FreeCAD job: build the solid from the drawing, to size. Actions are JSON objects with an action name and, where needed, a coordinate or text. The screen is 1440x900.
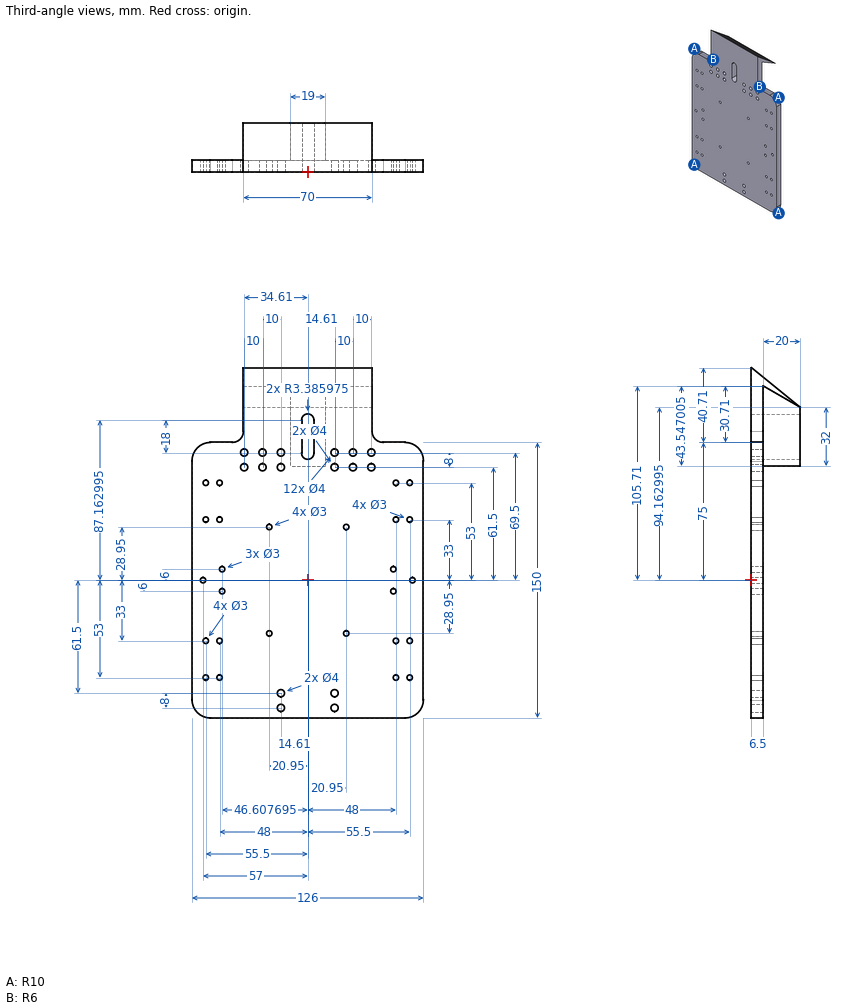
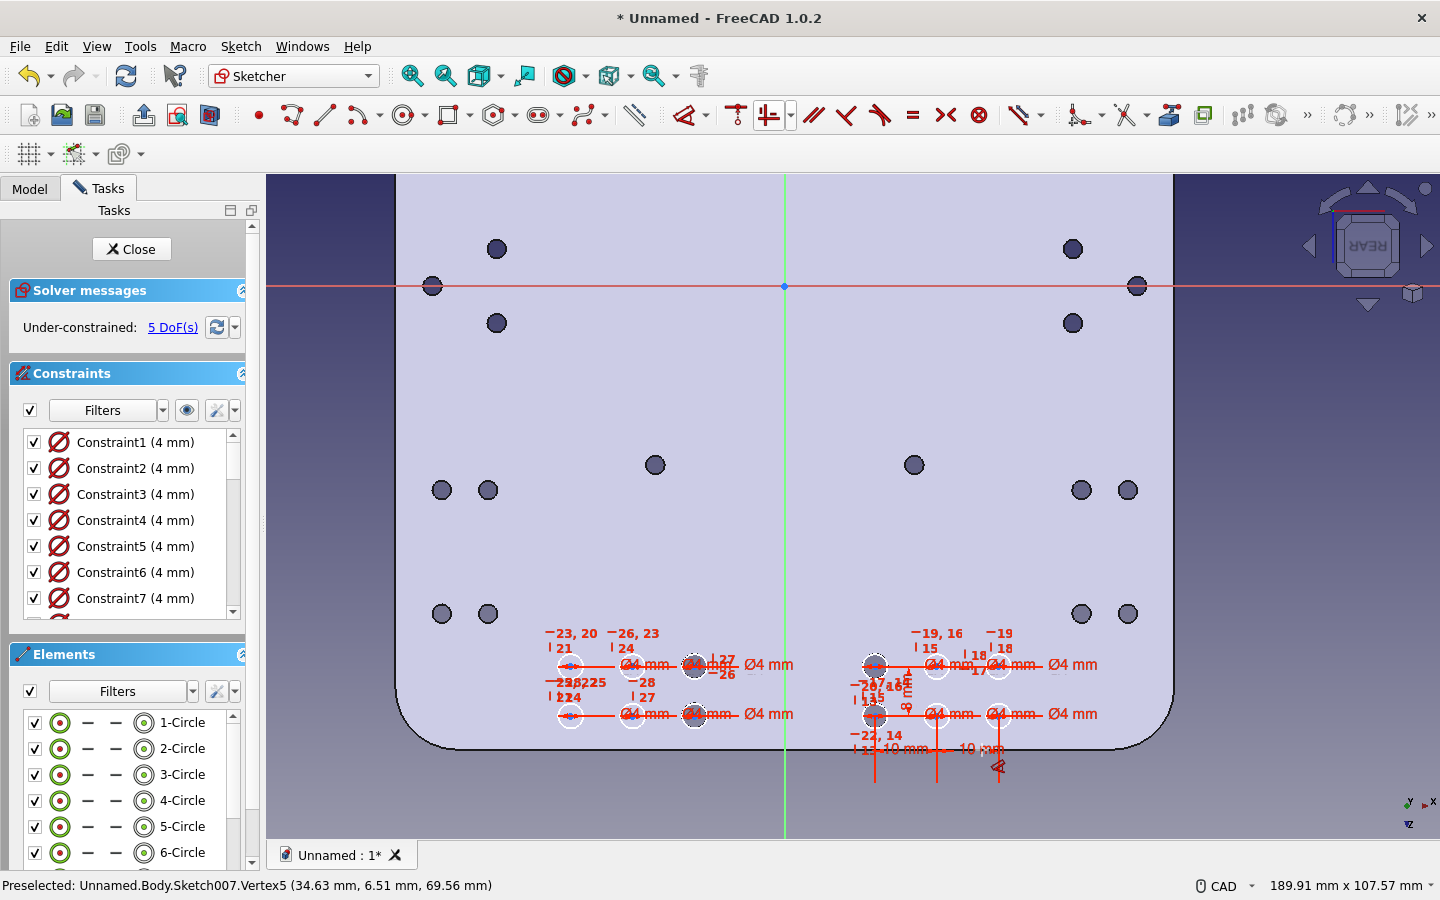
{"action": "left_click", "coordinate": [571, 667]}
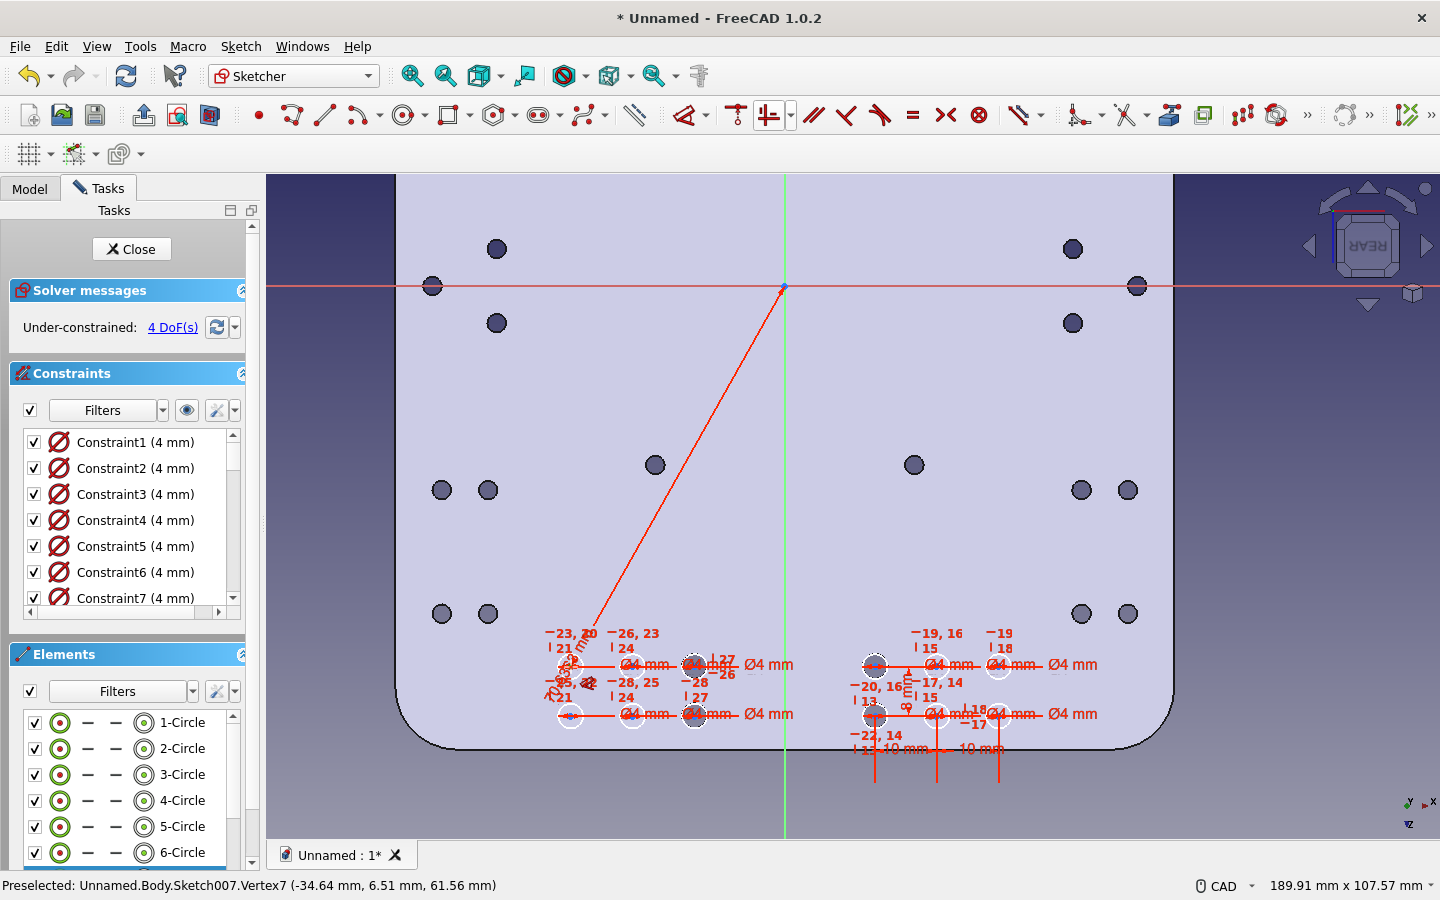
{"action": "left_click", "coordinate": [633, 667]}
{"action": "left_click", "coordinate": [602, 701]}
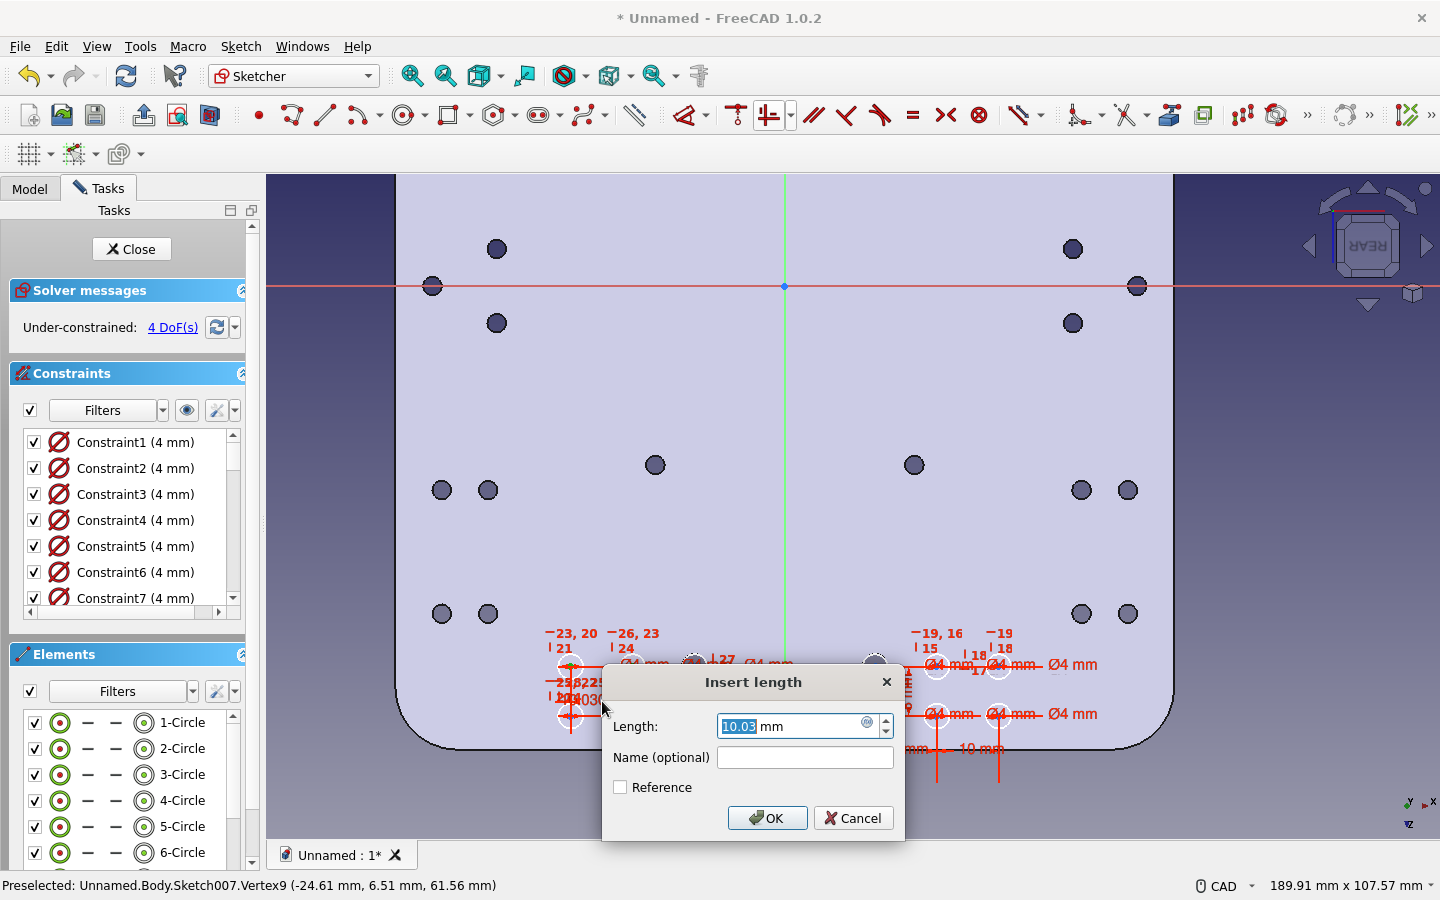
{"action": "type", "text": "10"}
{"action": "key", "text": "Return"}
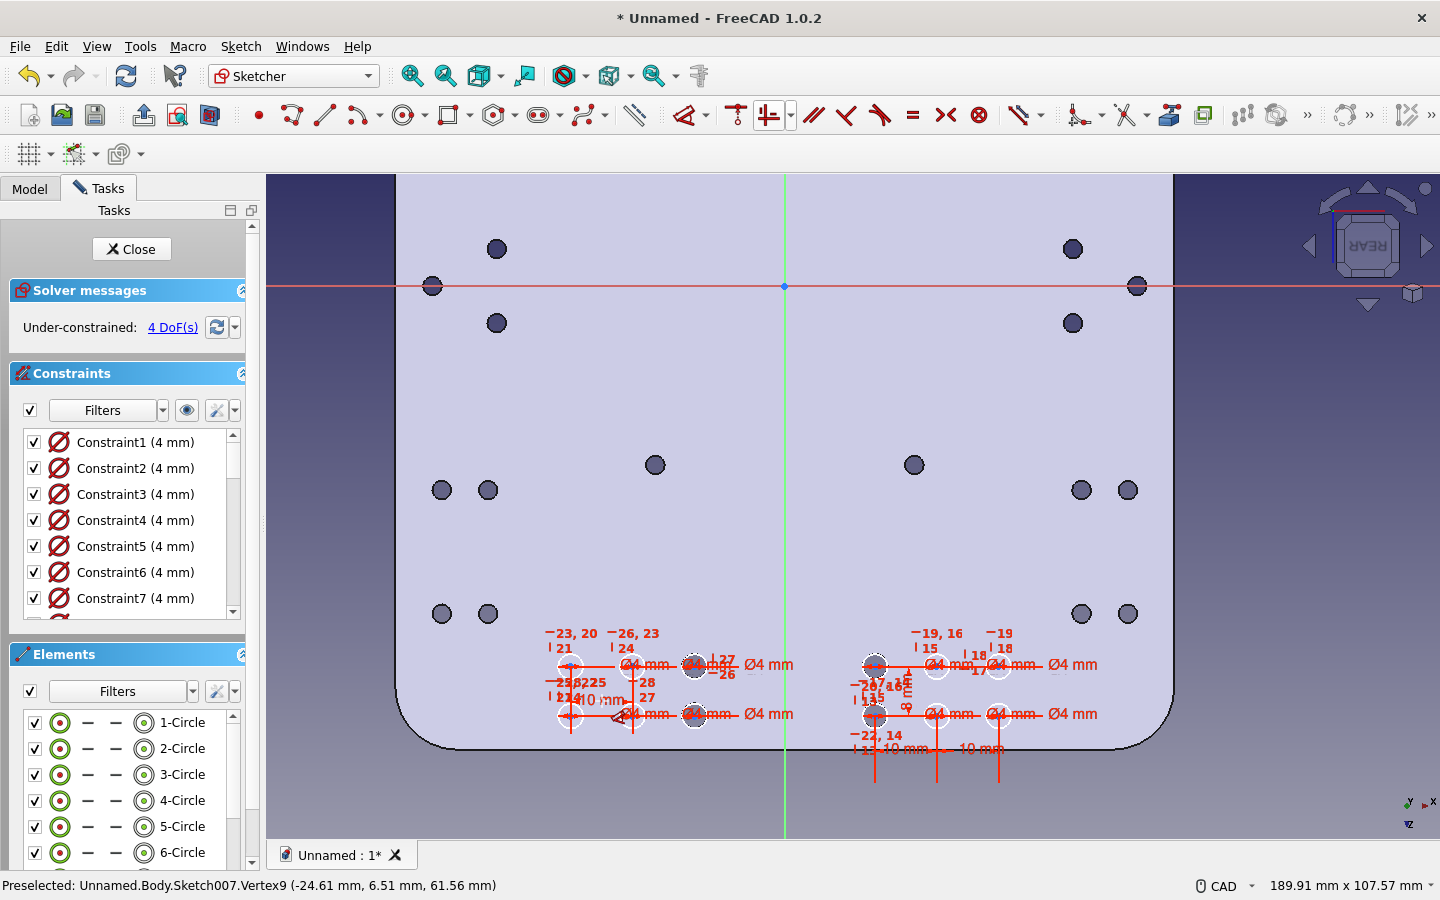
{"action": "left_click", "coordinate": [633, 667]}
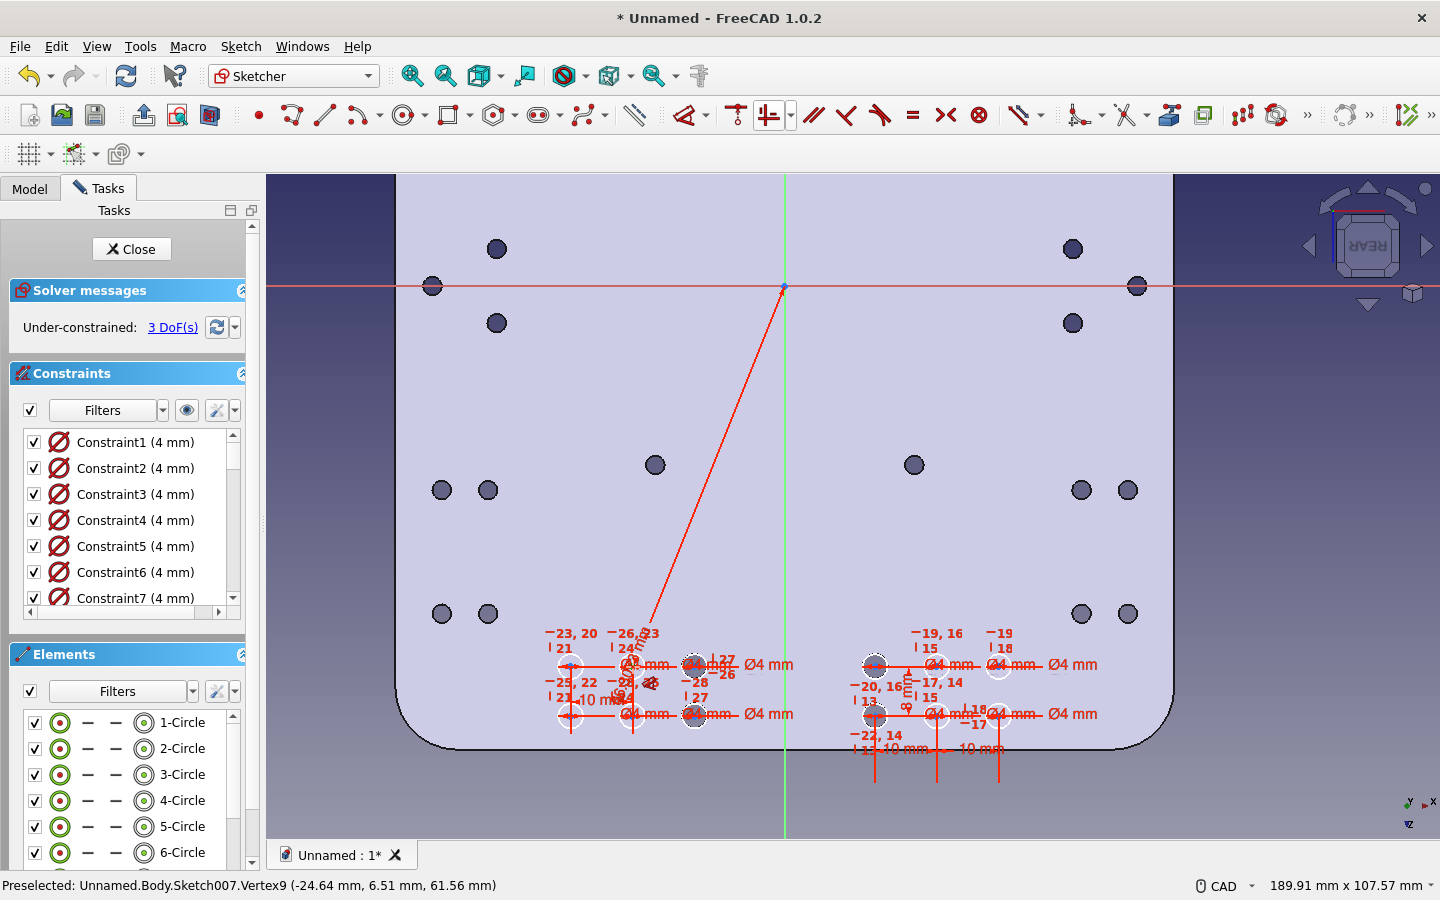
{"action": "left_click", "coordinate": [695, 667]}
{"action": "left_click", "coordinate": [664, 633]}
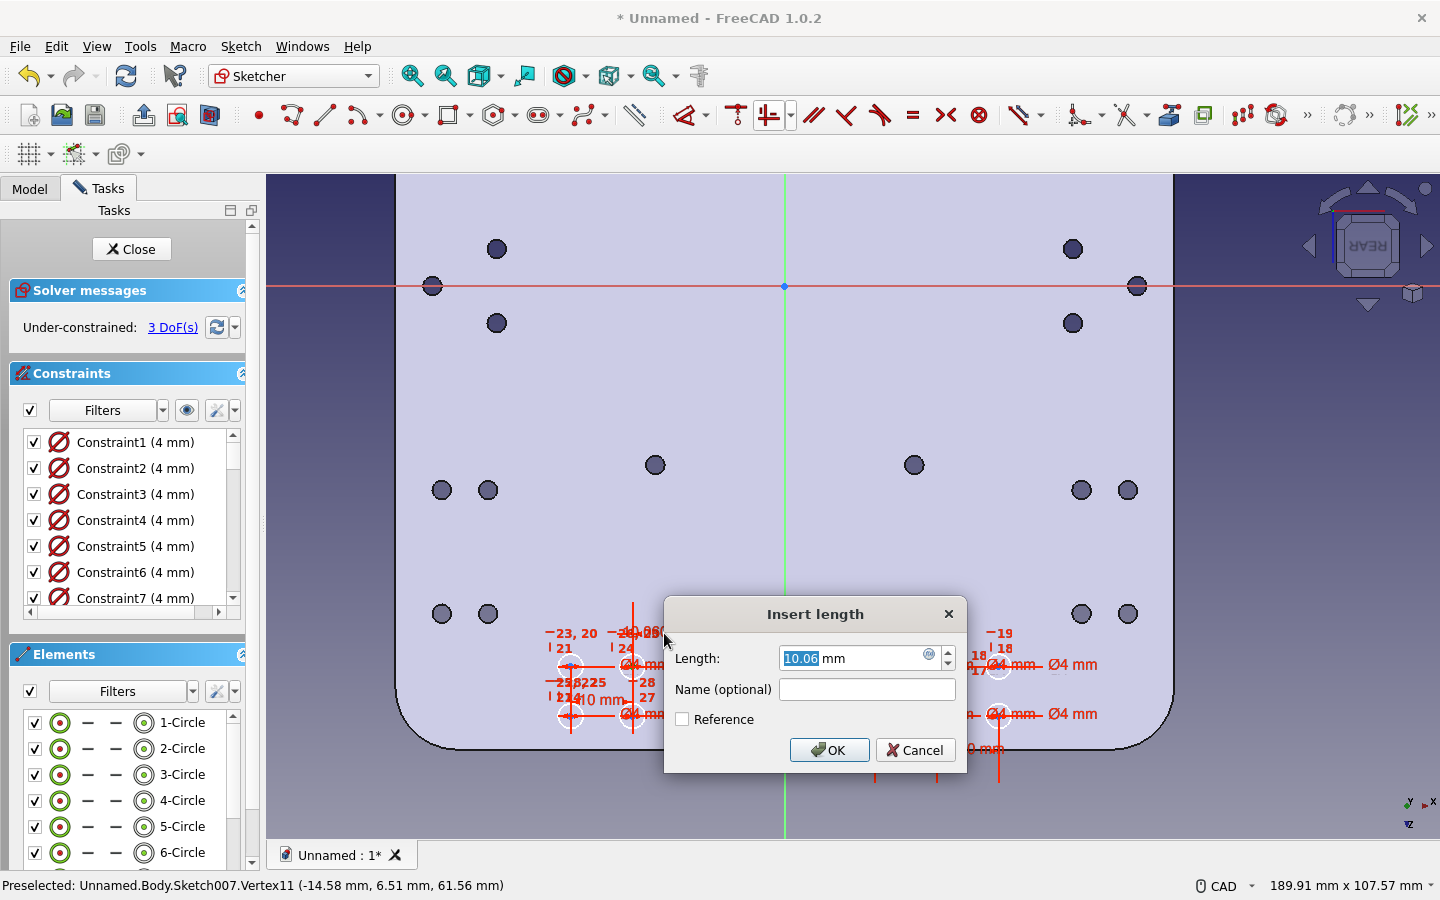
{"action": "type", "text": "10"}
{"action": "key", "text": "Return"}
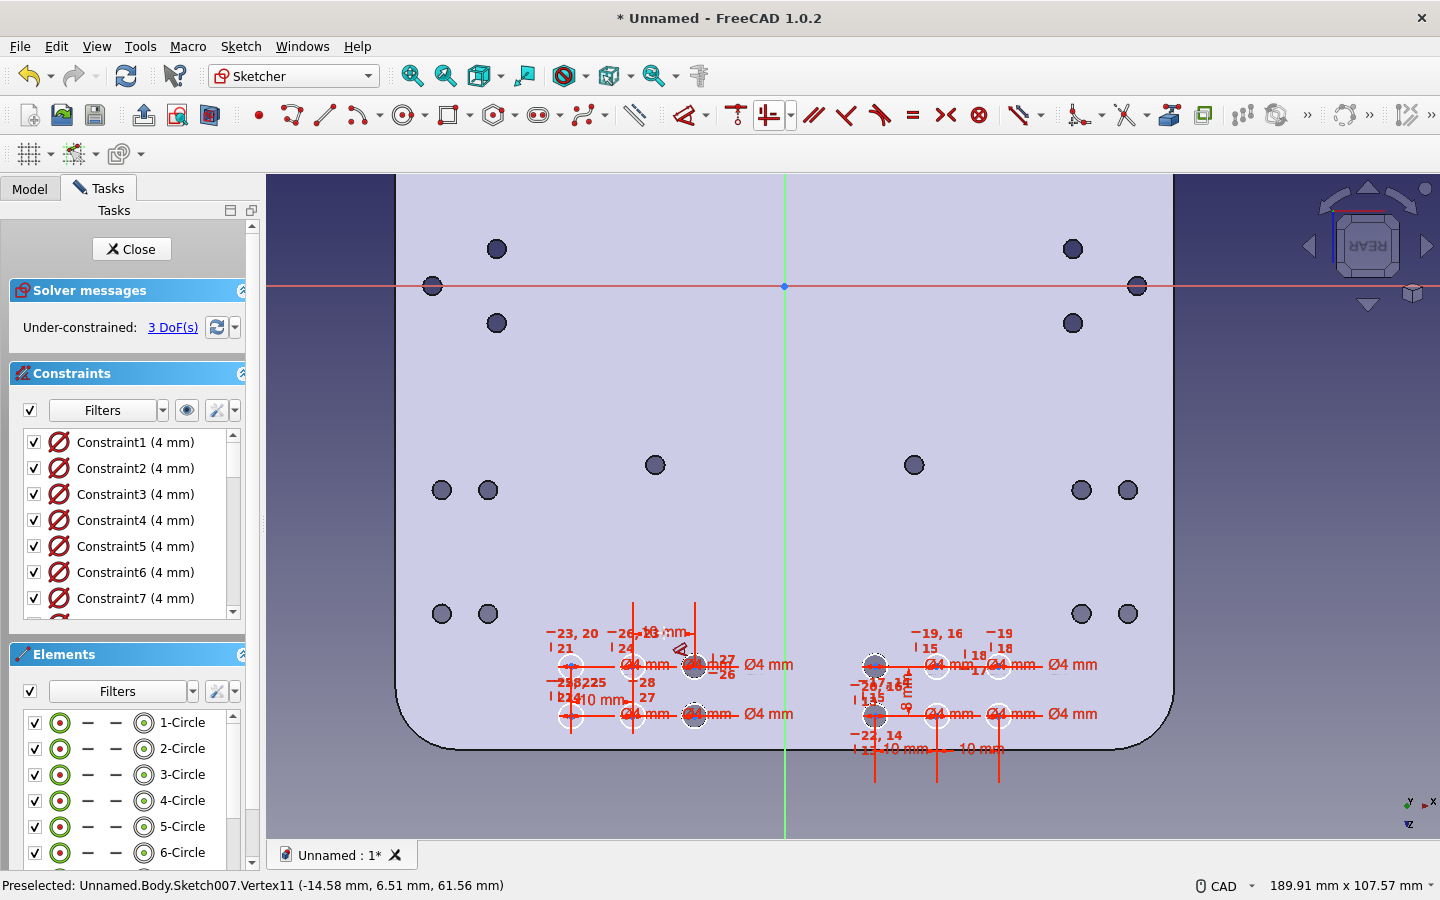
{"action": "left_click", "coordinate": [875, 716]}
{"action": "left_click", "coordinate": [909, 501]}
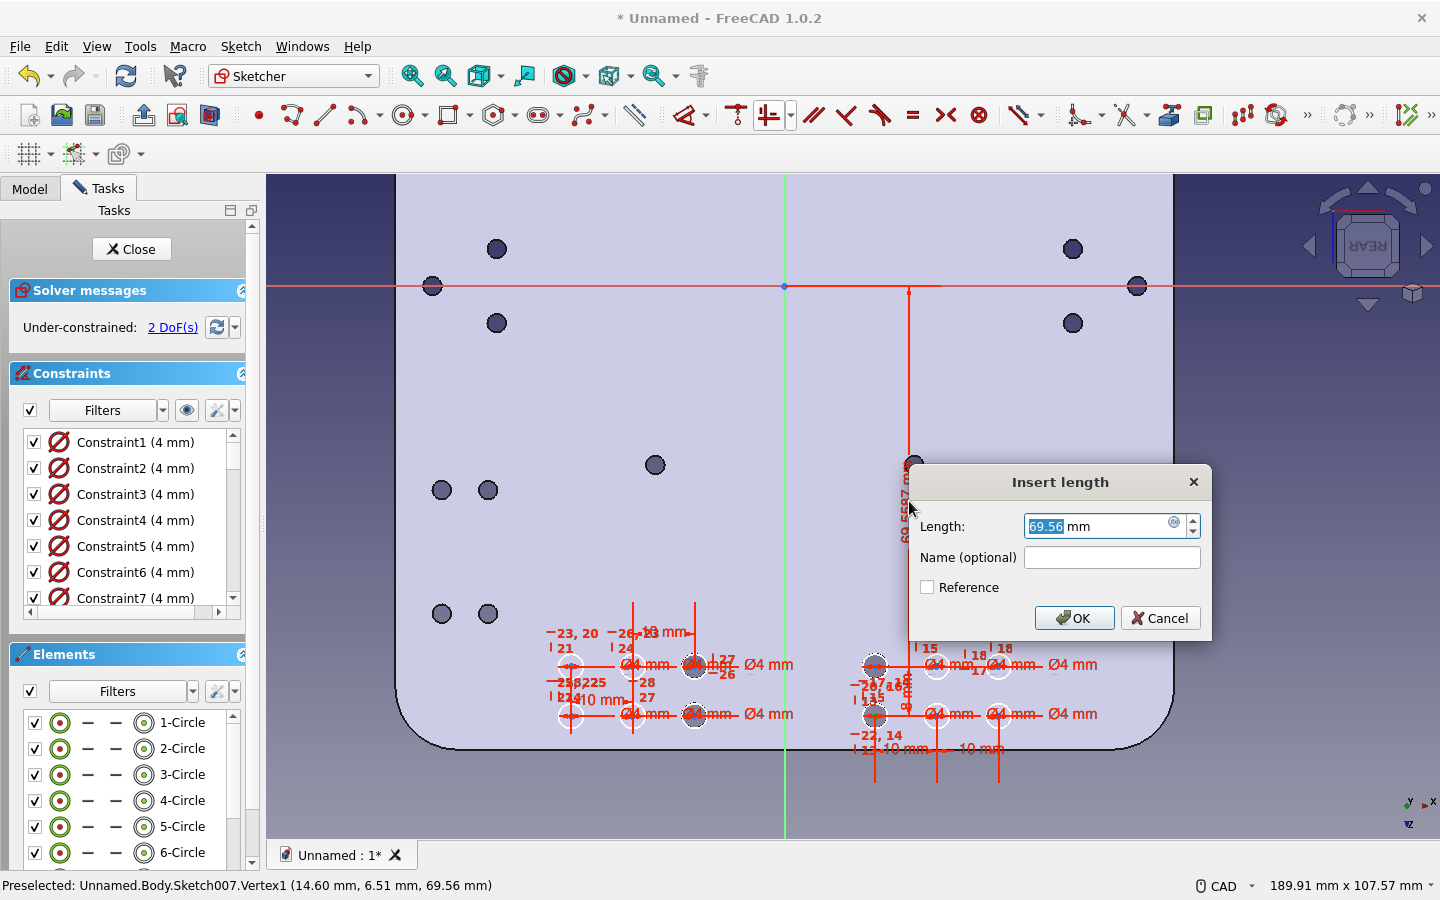
{"action": "type", "text": "69.5"}
{"action": "key", "text": "Return"}